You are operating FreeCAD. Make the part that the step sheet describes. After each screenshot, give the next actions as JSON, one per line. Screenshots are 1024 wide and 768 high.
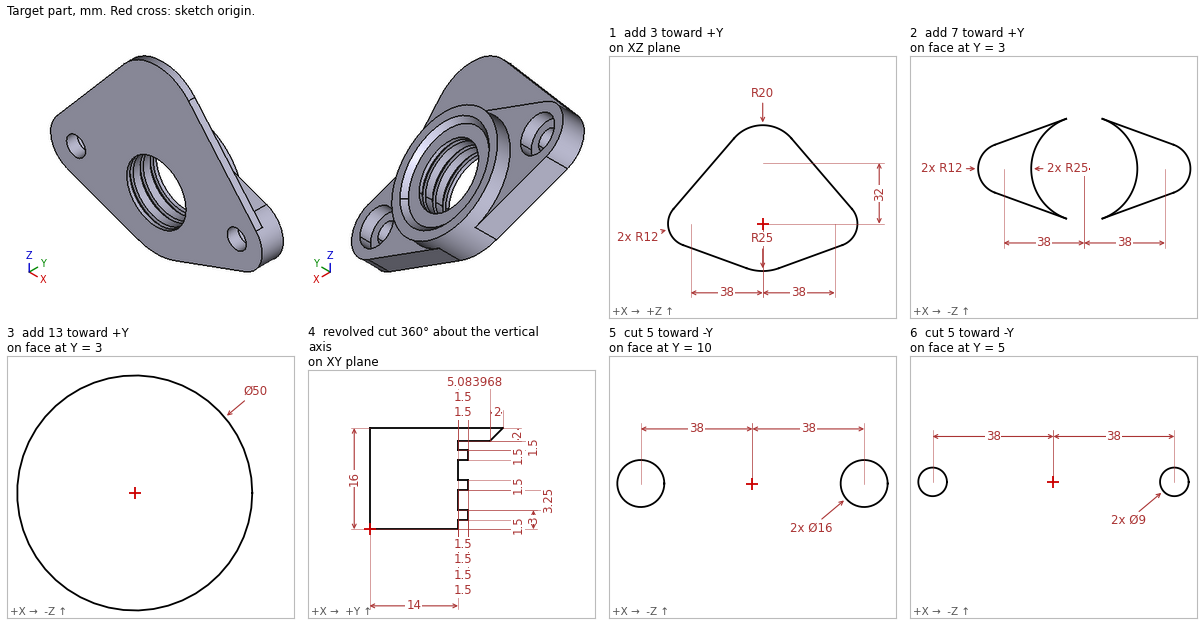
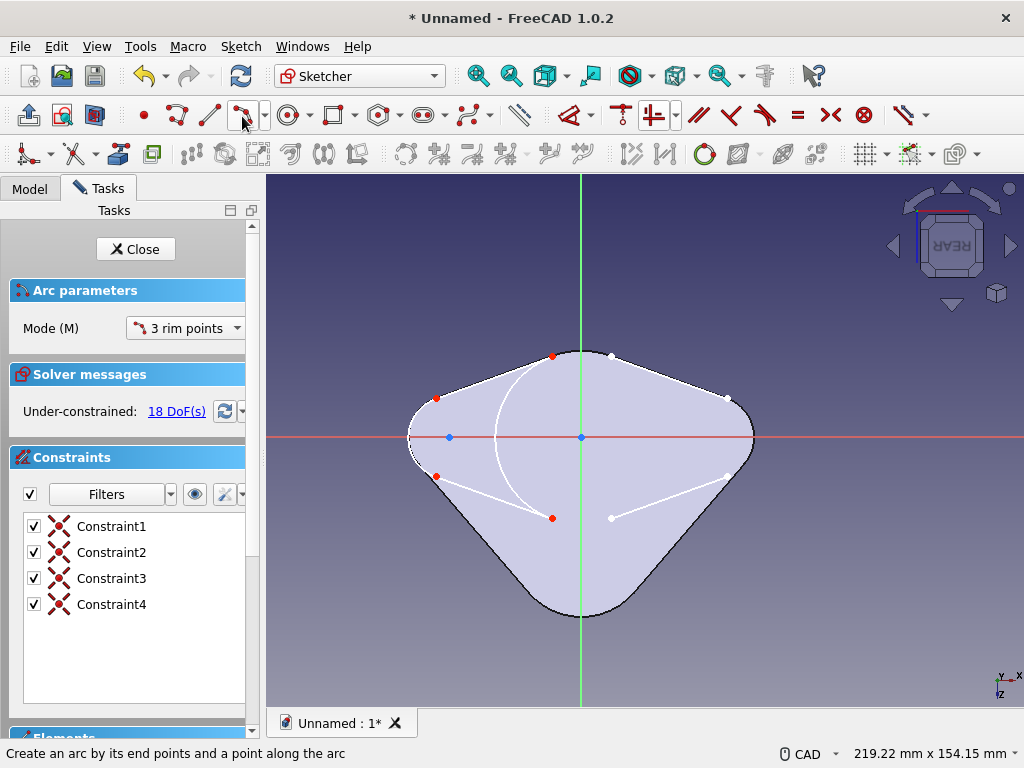
{"action": "left_click", "coordinate": [727, 477]}
{"action": "left_click", "coordinate": [727, 399]}
{"action": "left_click", "coordinate": [749, 457]}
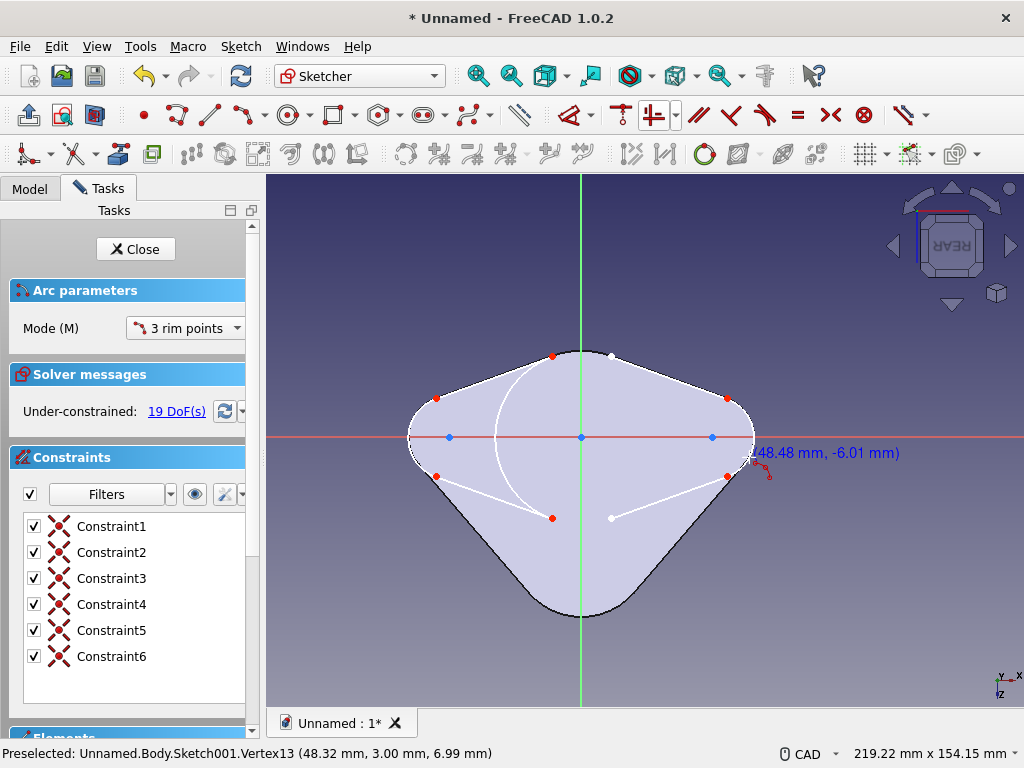
{"action": "left_click", "coordinate": [611, 357]}
{"action": "left_click", "coordinate": [611, 519]}
{"action": "left_click", "coordinate": [665, 458]}
{"action": "key", "text": "Escape"}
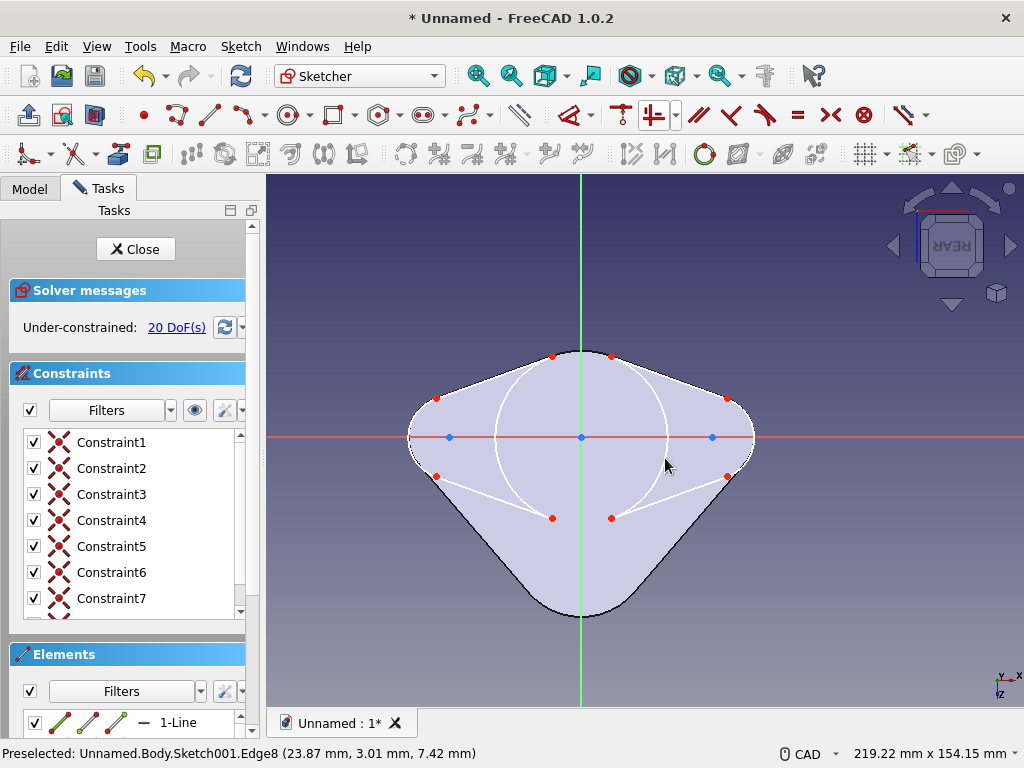
{"action": "left_click", "coordinate": [471, 490]}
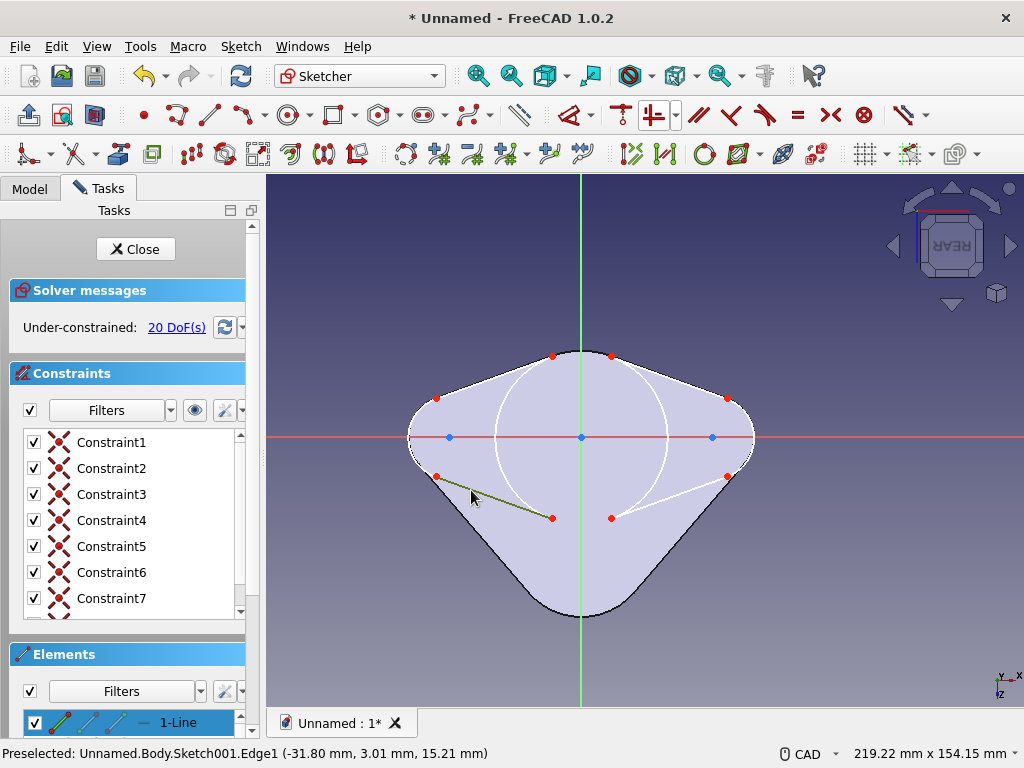
{"action": "left_click", "coordinate": [505, 398]}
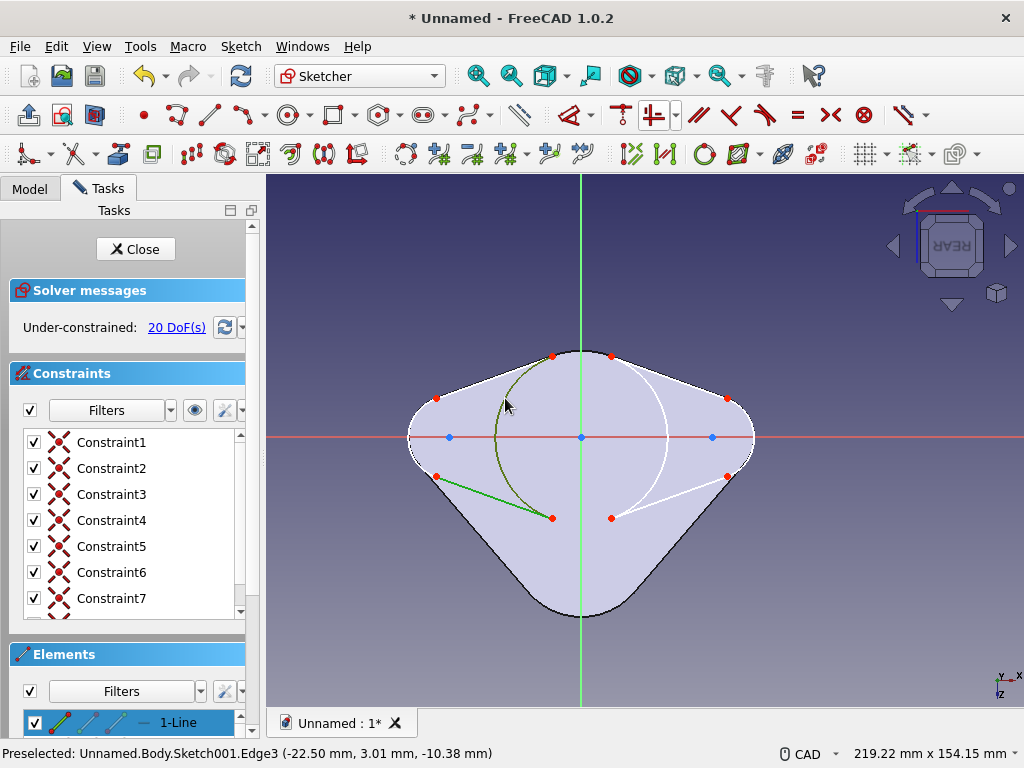
{"action": "left_click", "coordinate": [765, 116]}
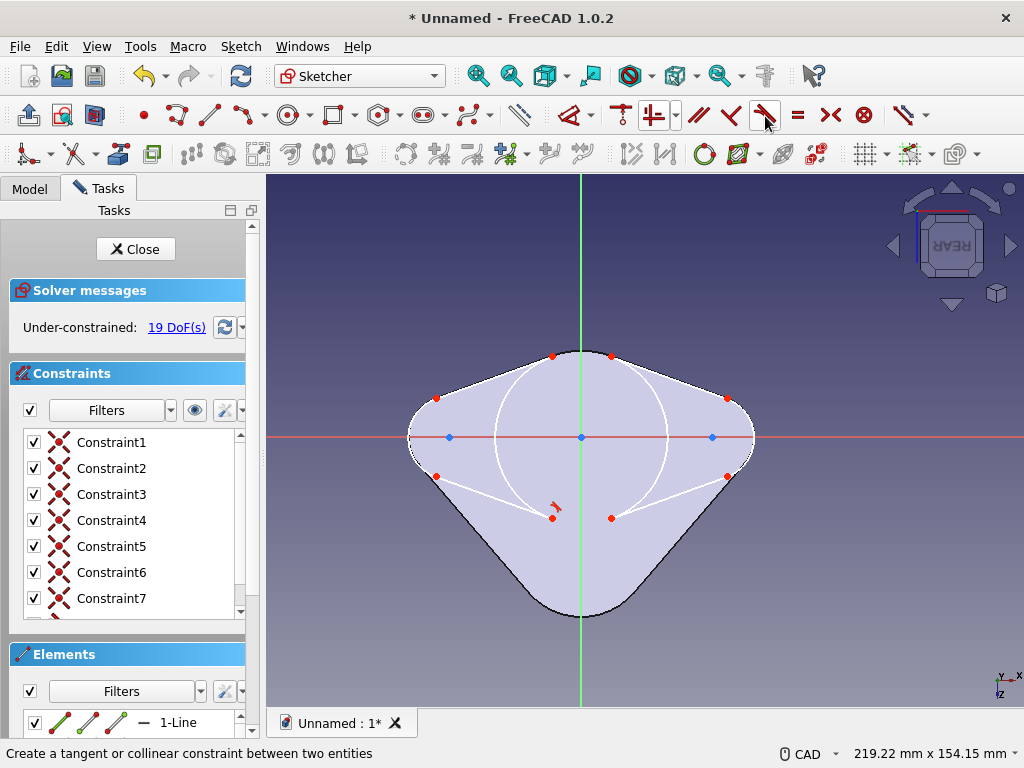
{"action": "left_click", "coordinate": [471, 490]}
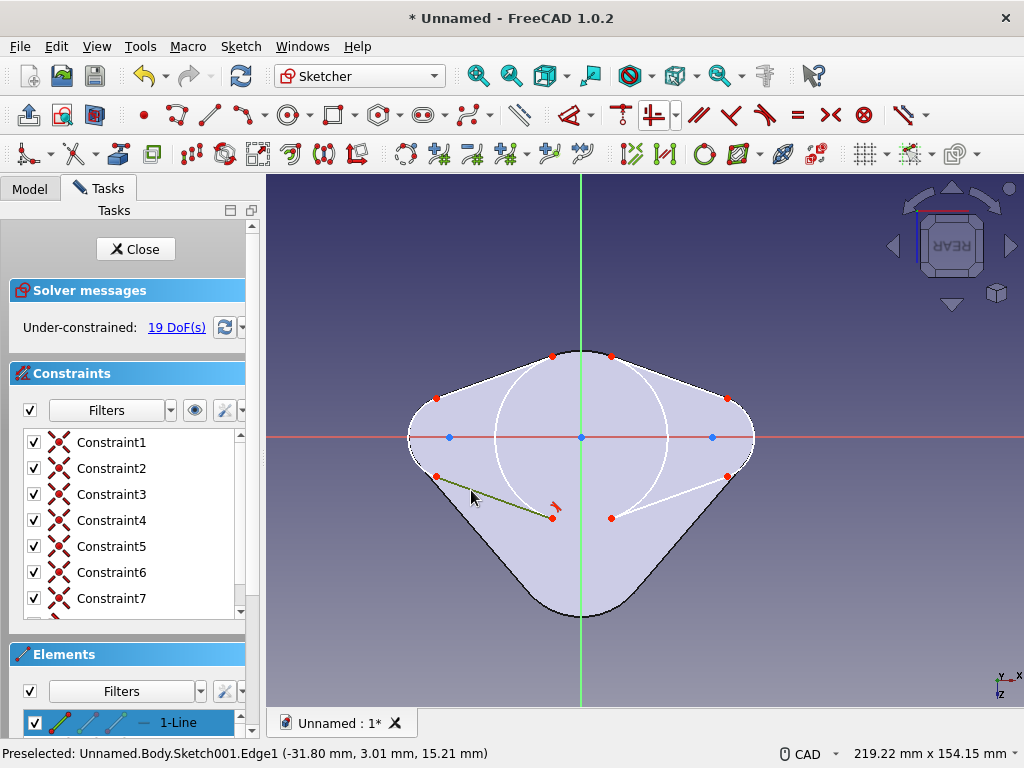
{"action": "left_click", "coordinate": [413, 418]}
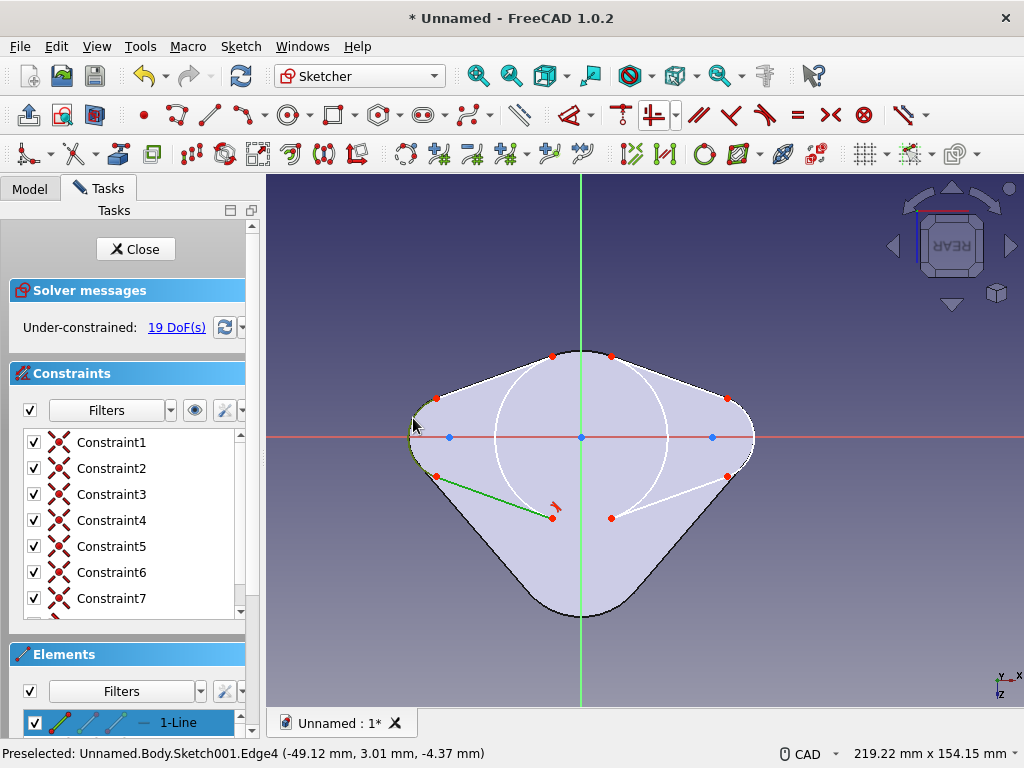
{"action": "left_click", "coordinate": [765, 116]}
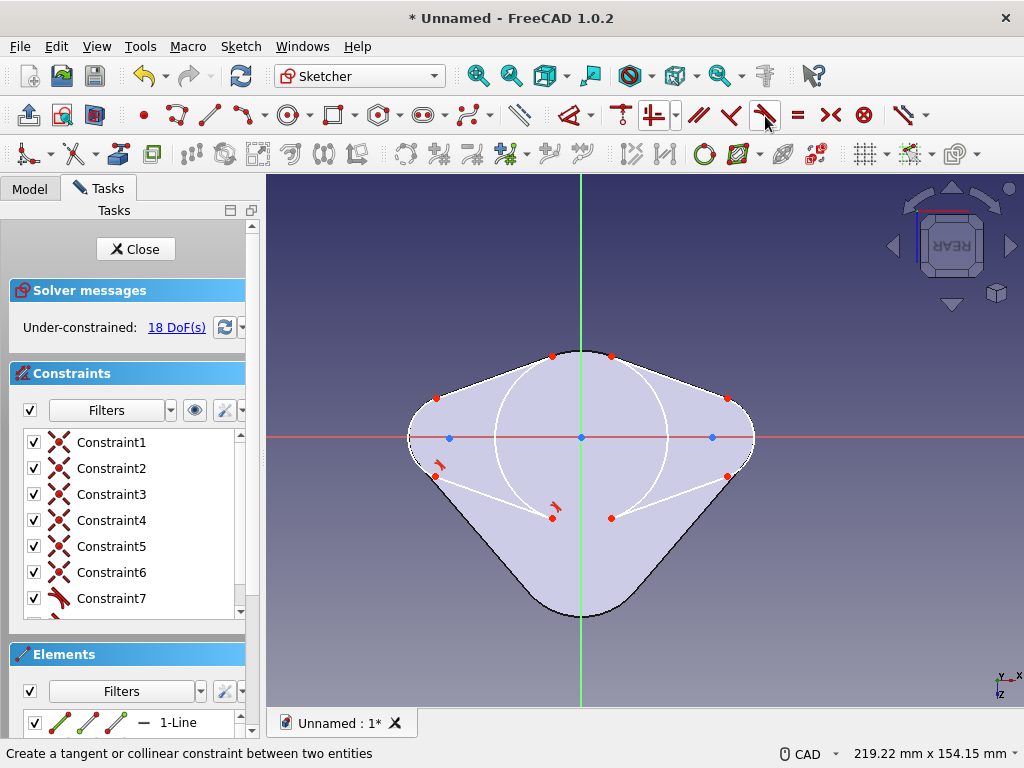
{"action": "left_click", "coordinate": [471, 386]}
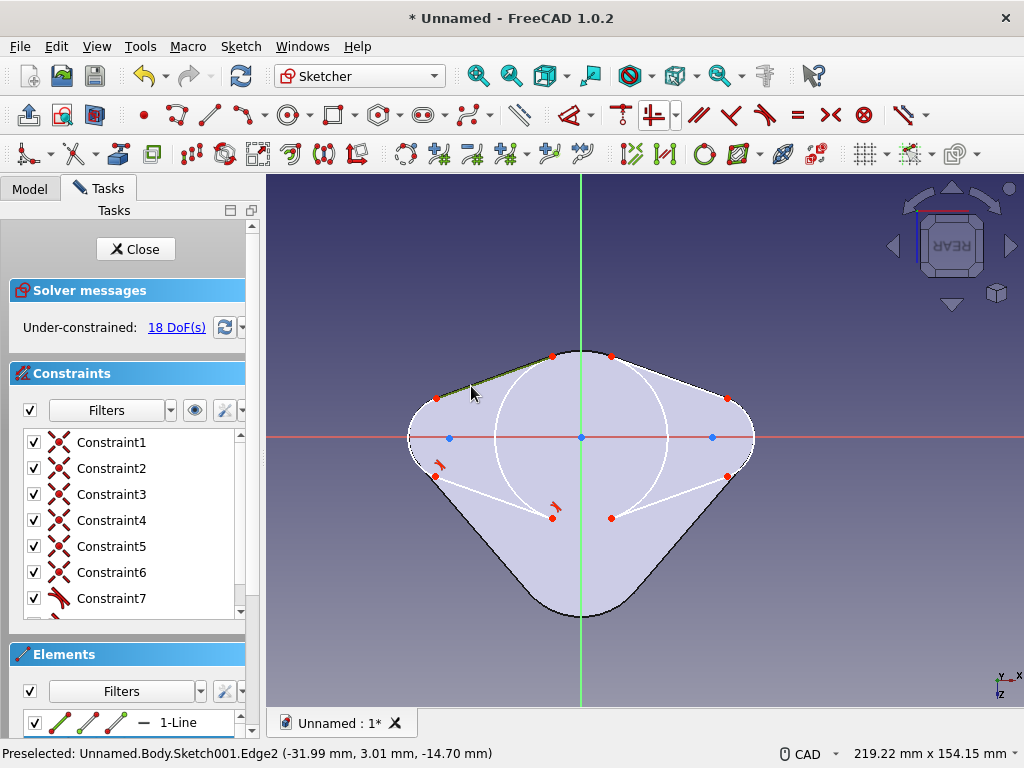
{"action": "left_click", "coordinate": [505, 397]}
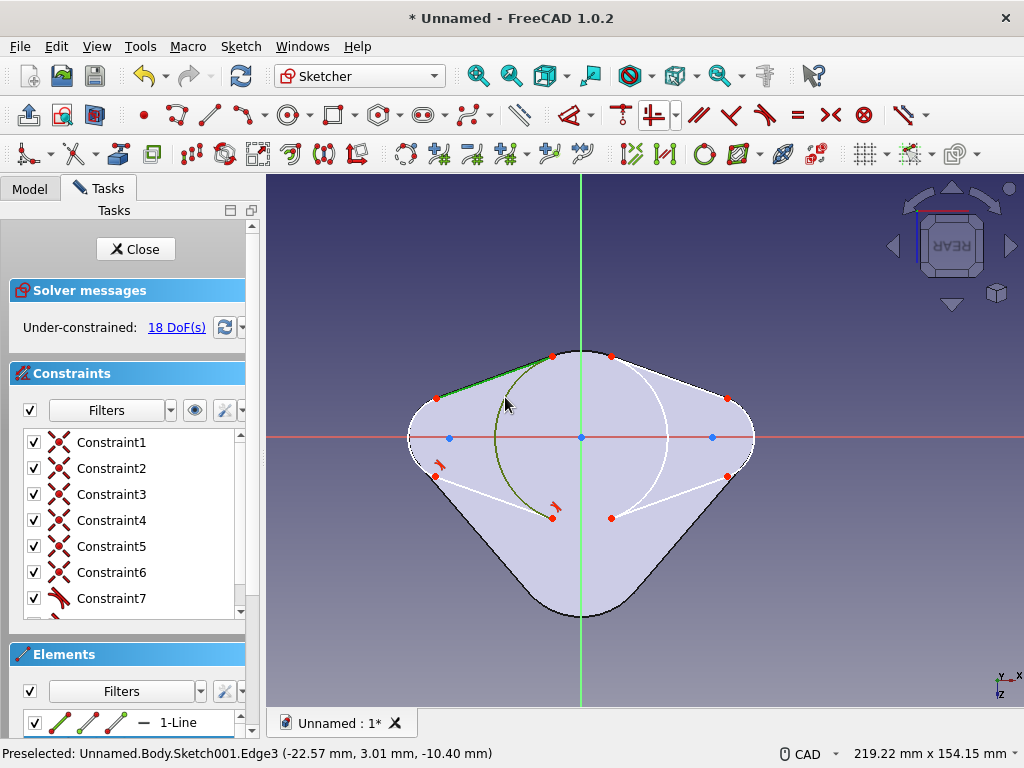
{"action": "left_click", "coordinate": [765, 116]}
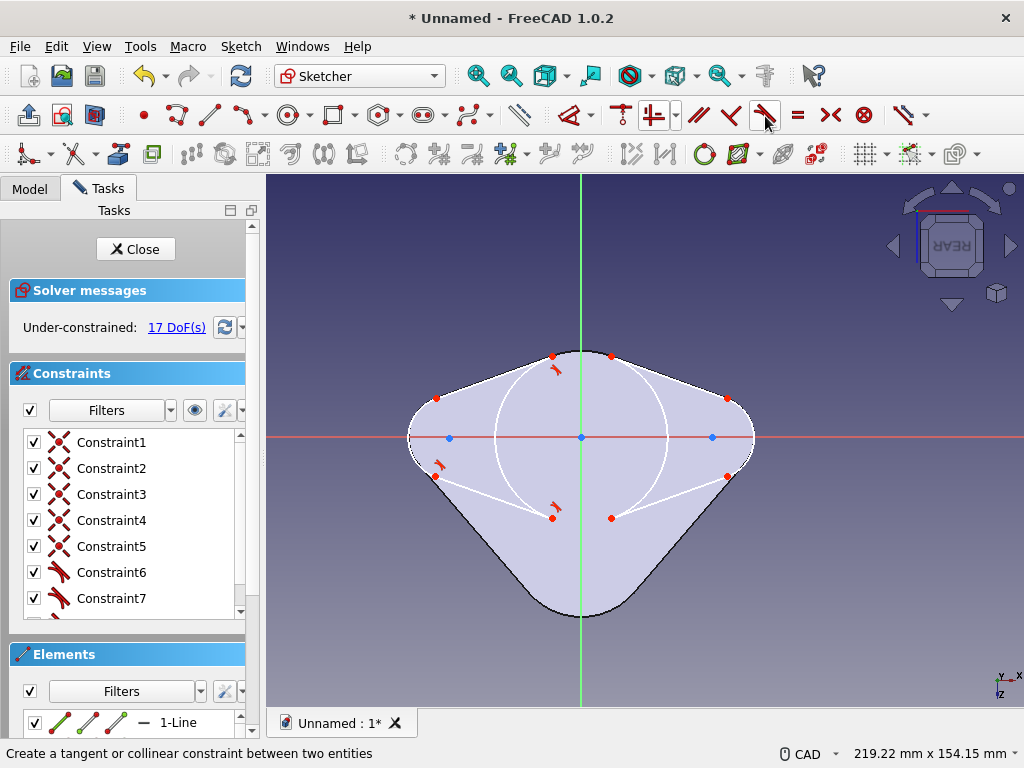
{"action": "left_click", "coordinate": [471, 386]}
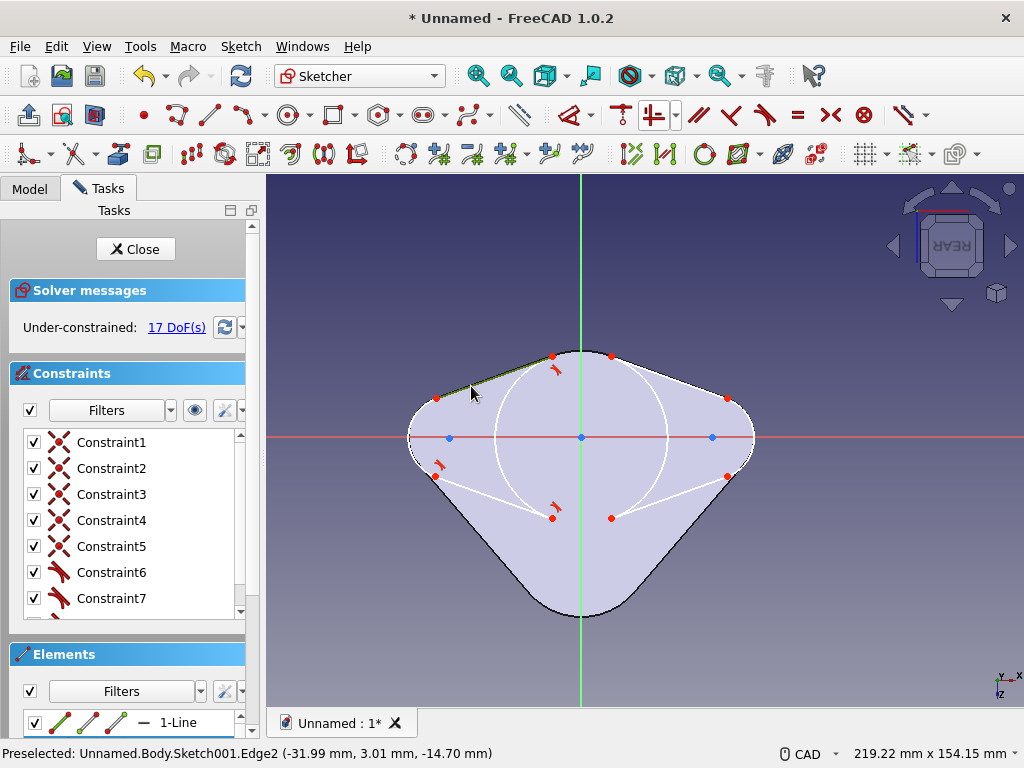
{"action": "left_click", "coordinate": [413, 418]}